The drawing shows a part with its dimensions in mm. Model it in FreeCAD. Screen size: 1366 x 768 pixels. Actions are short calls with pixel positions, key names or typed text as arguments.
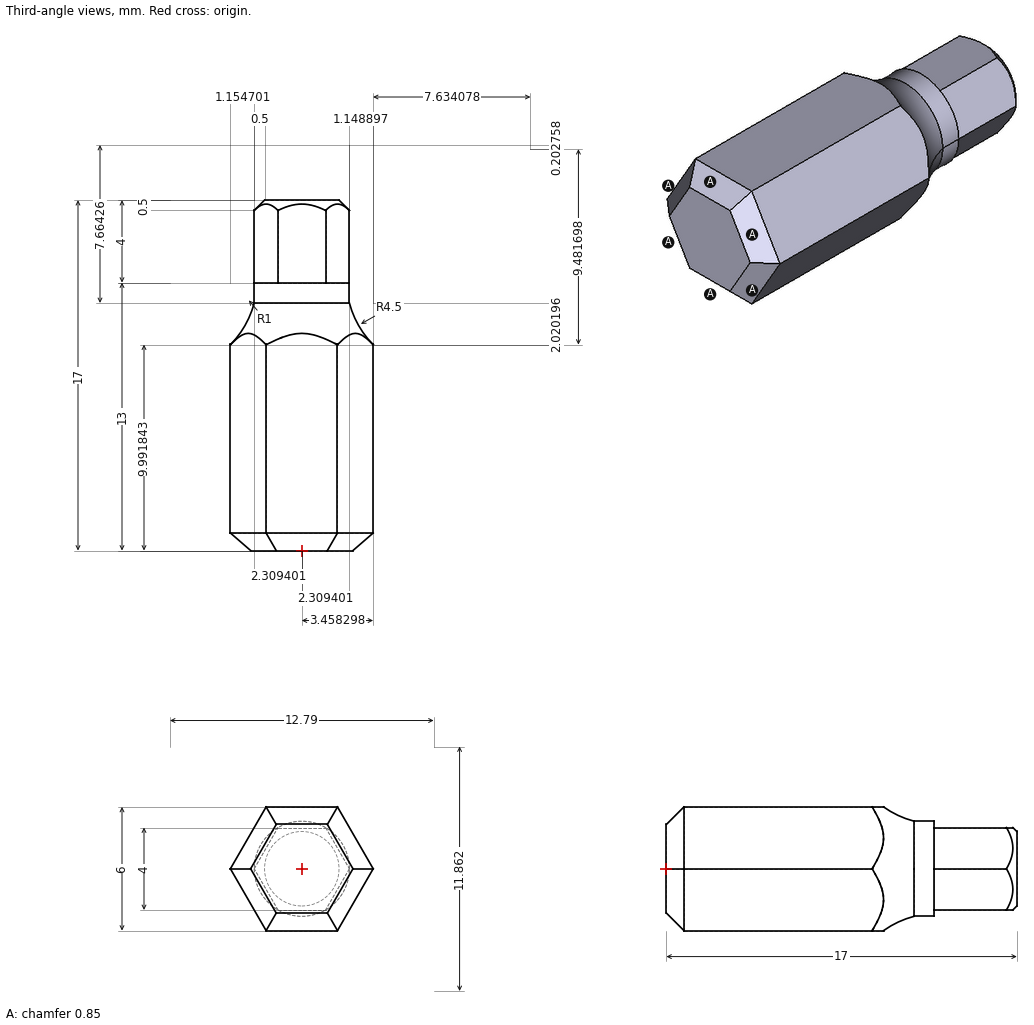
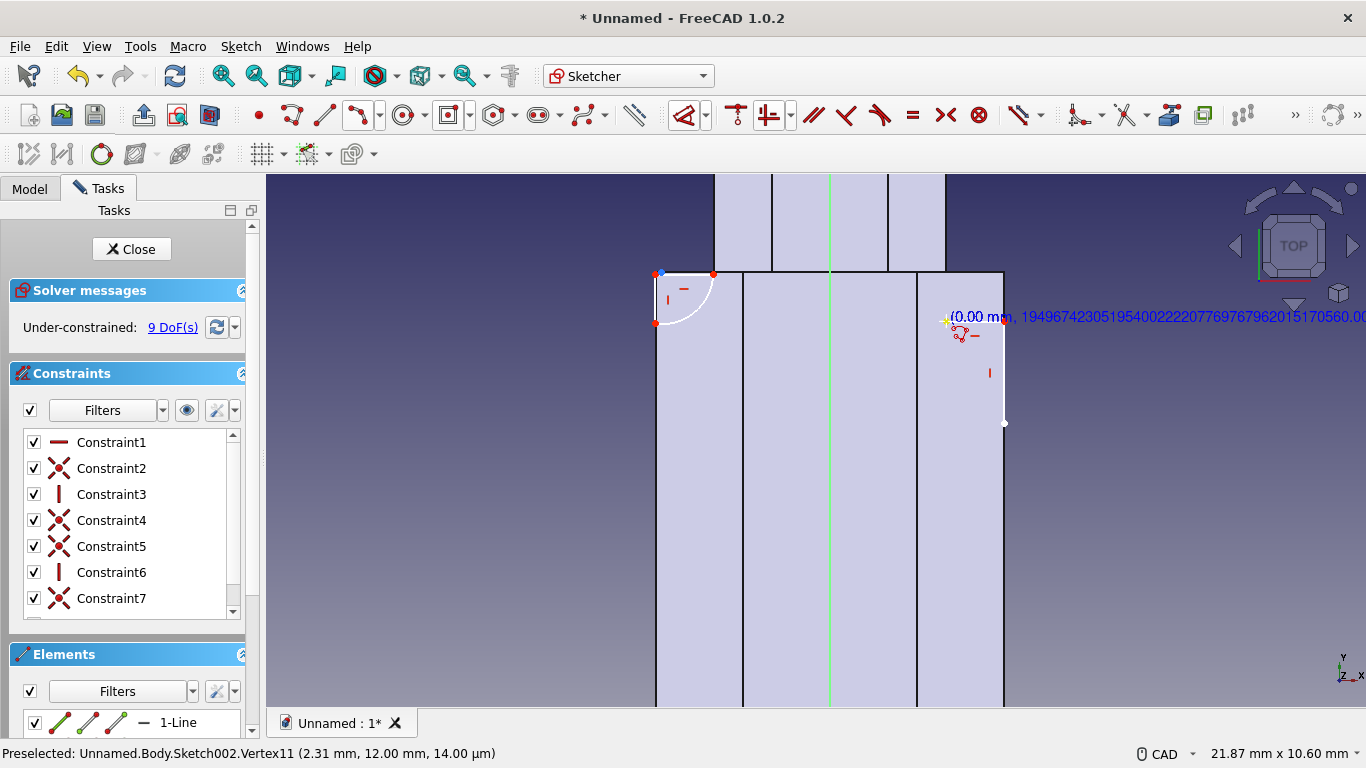
click(358, 116)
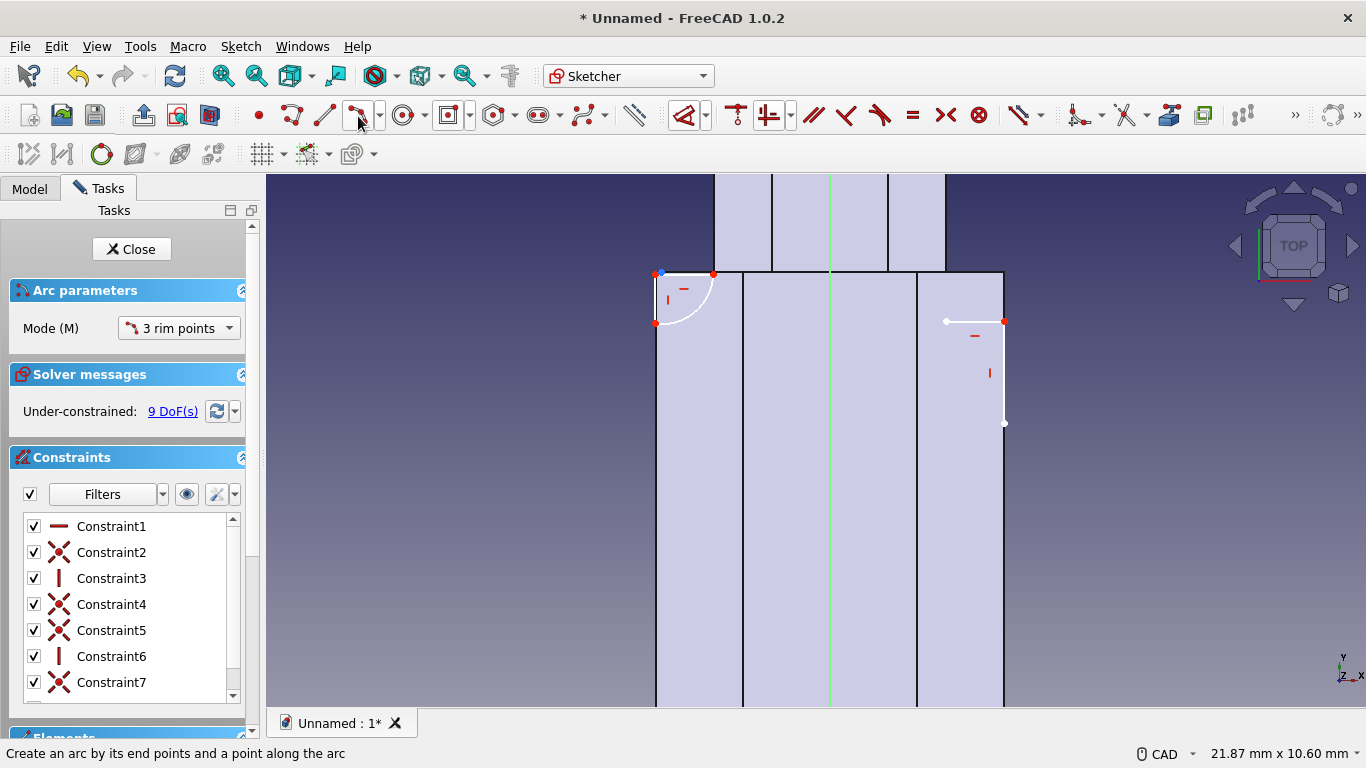
click(946, 322)
click(1004, 424)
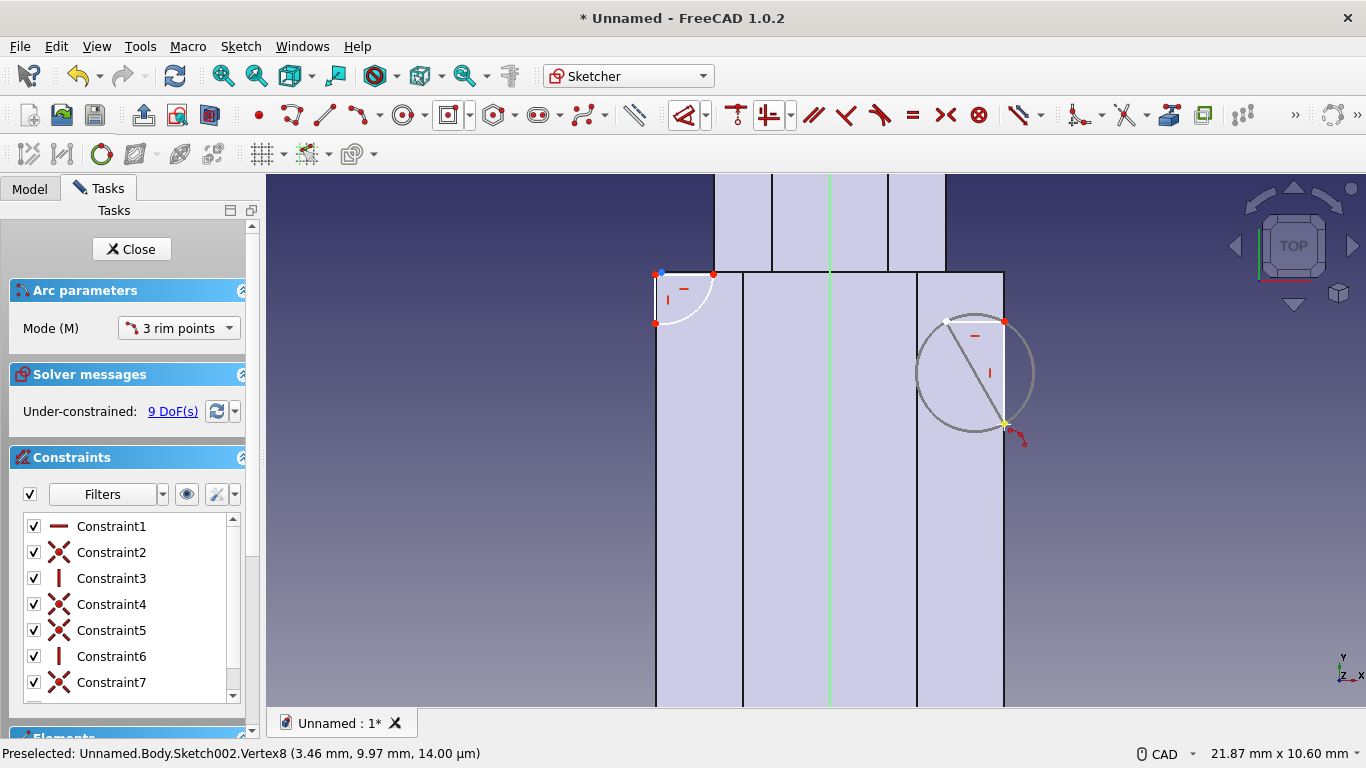
scroll(968, 376, up, 4)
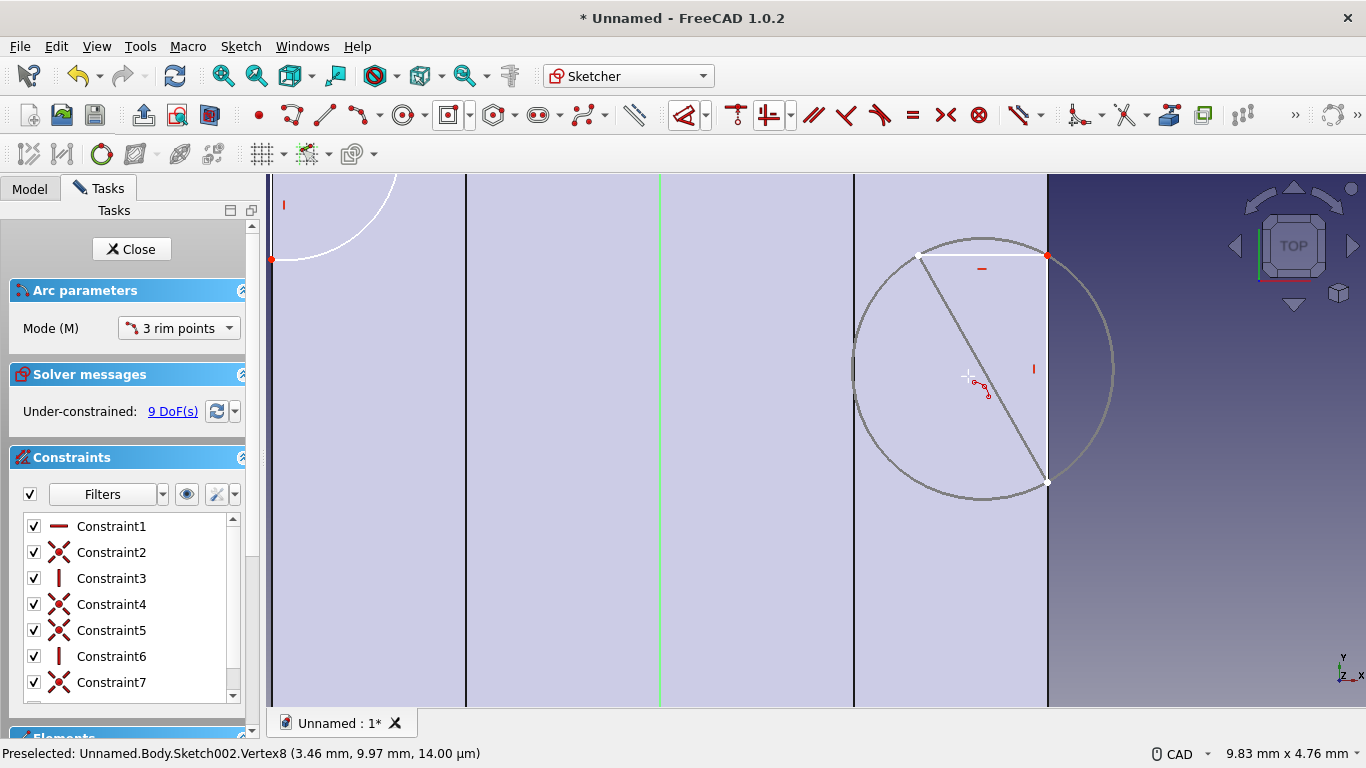
click(968, 376)
key(Escape)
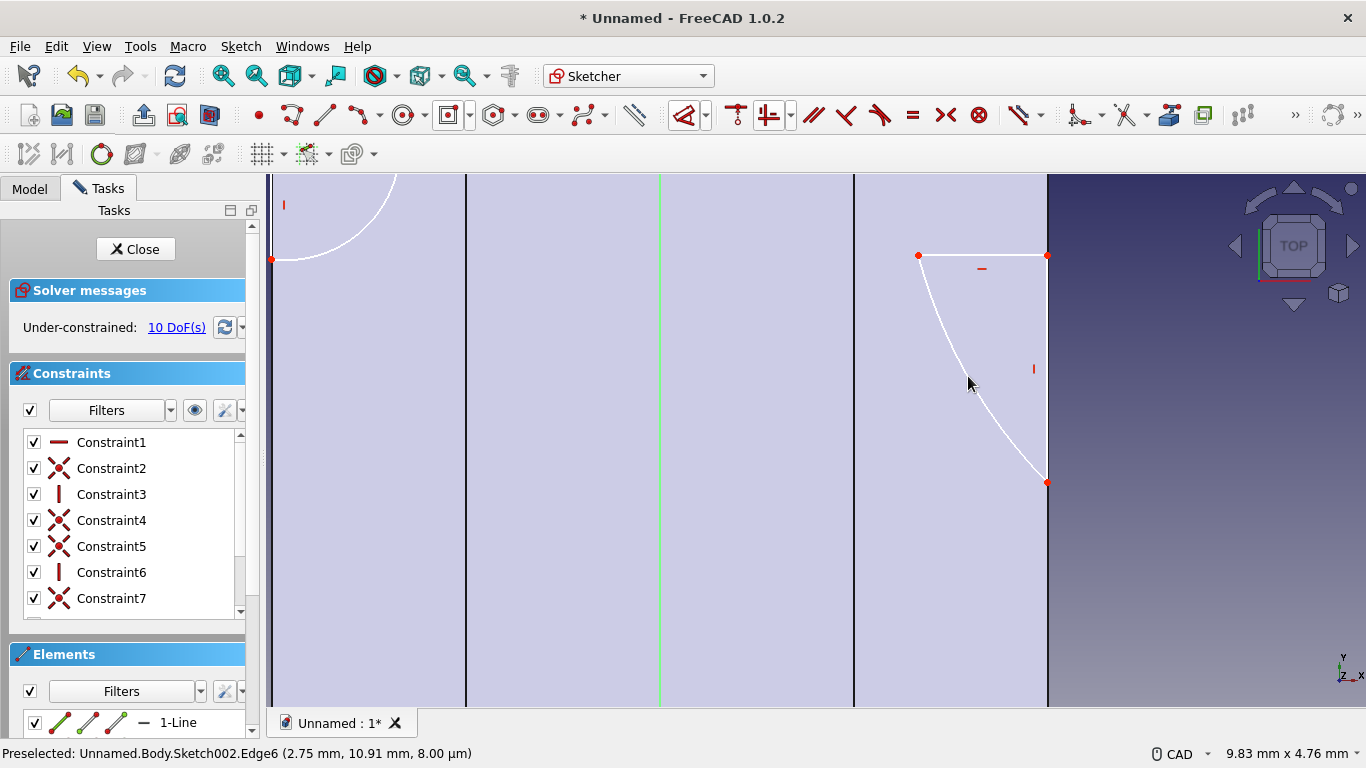
click(327, 252)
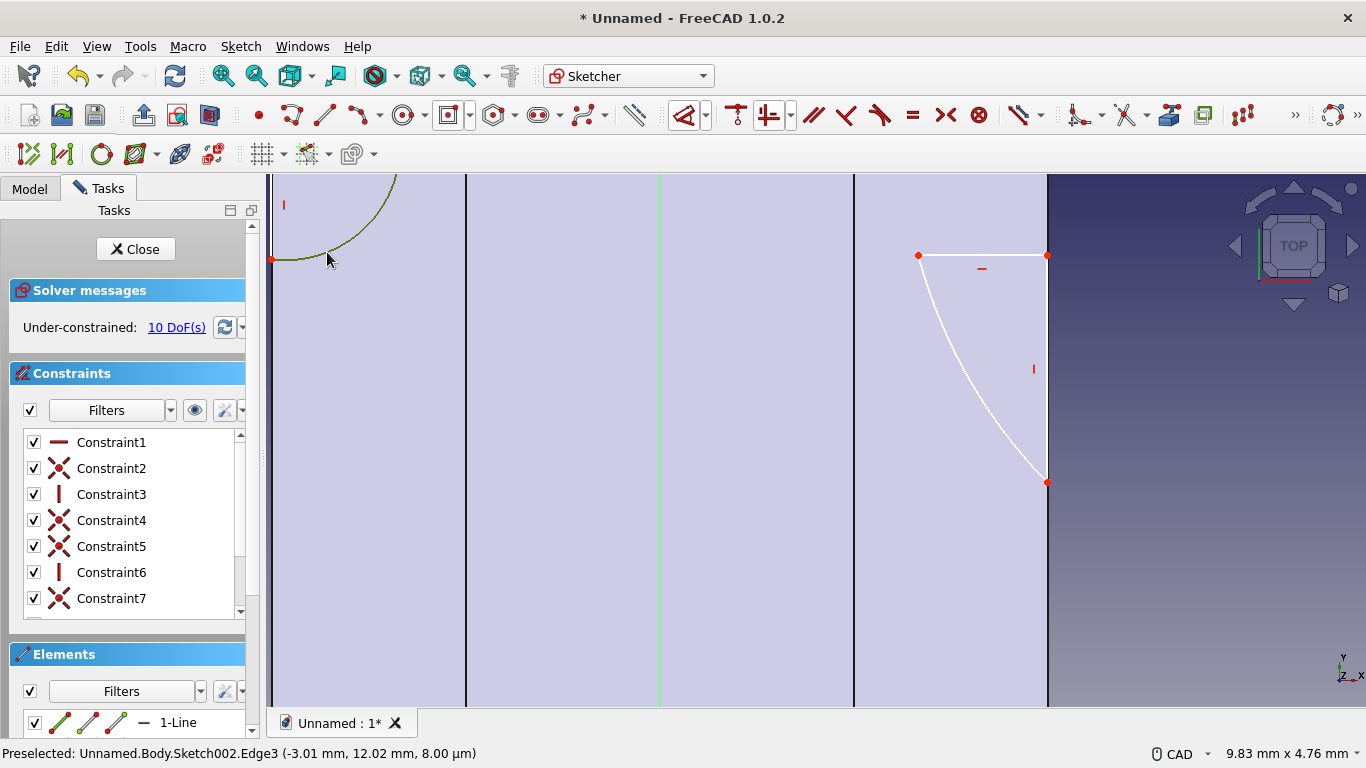
click(706, 116)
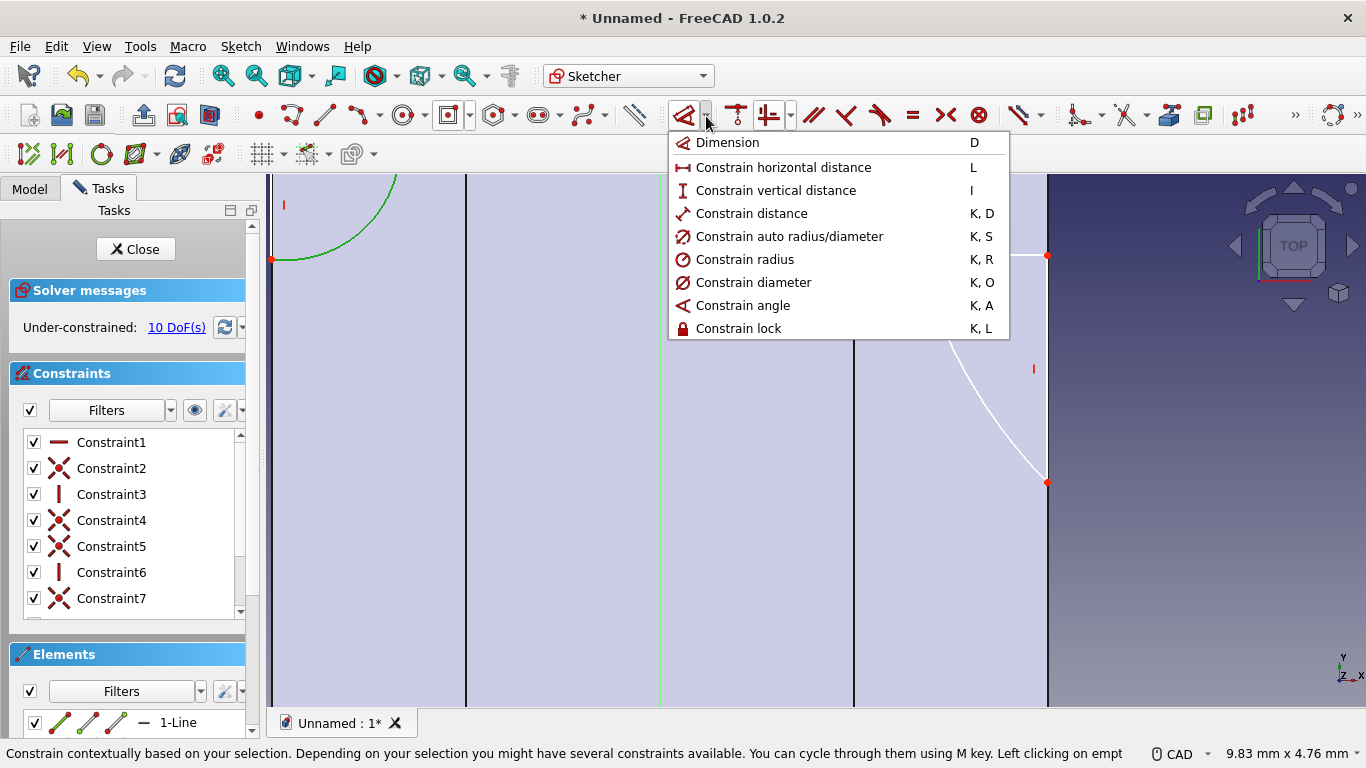
click(839, 260)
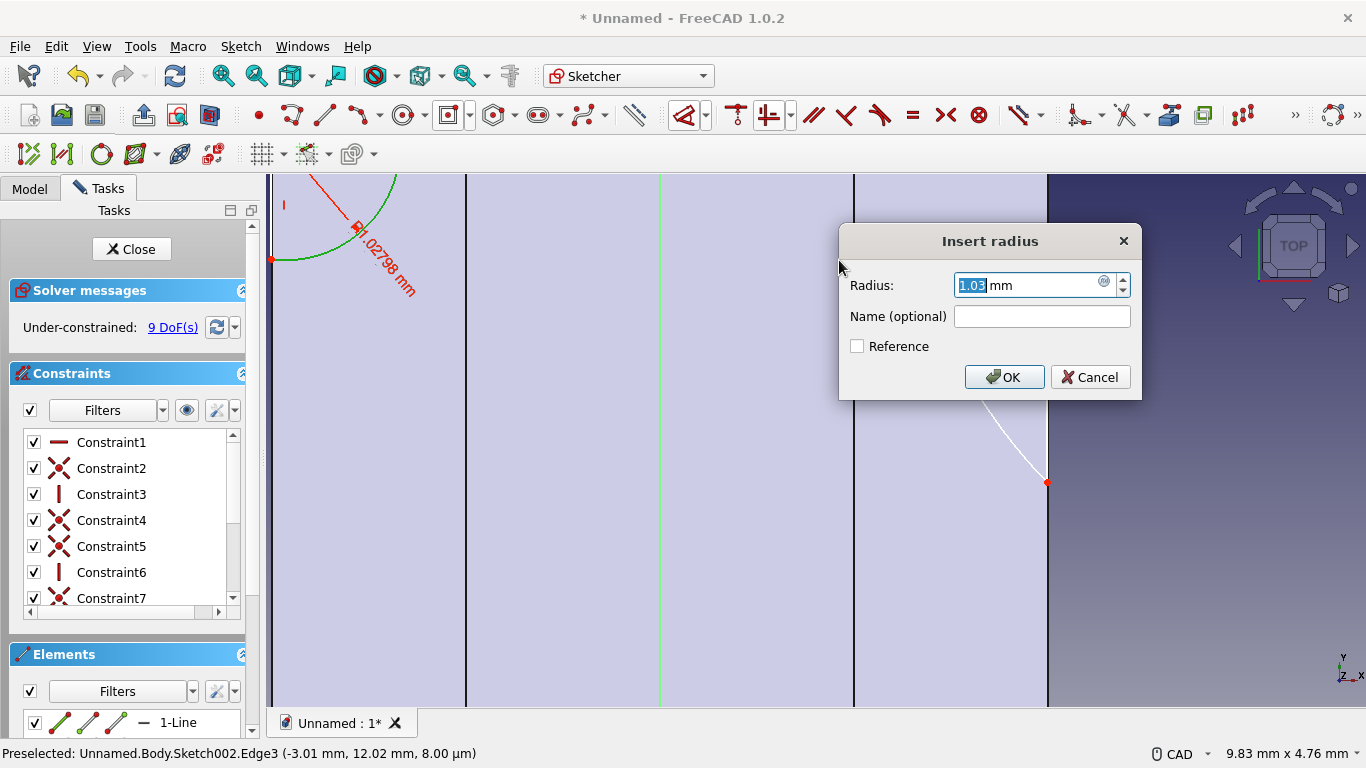
text(1)
key(Return)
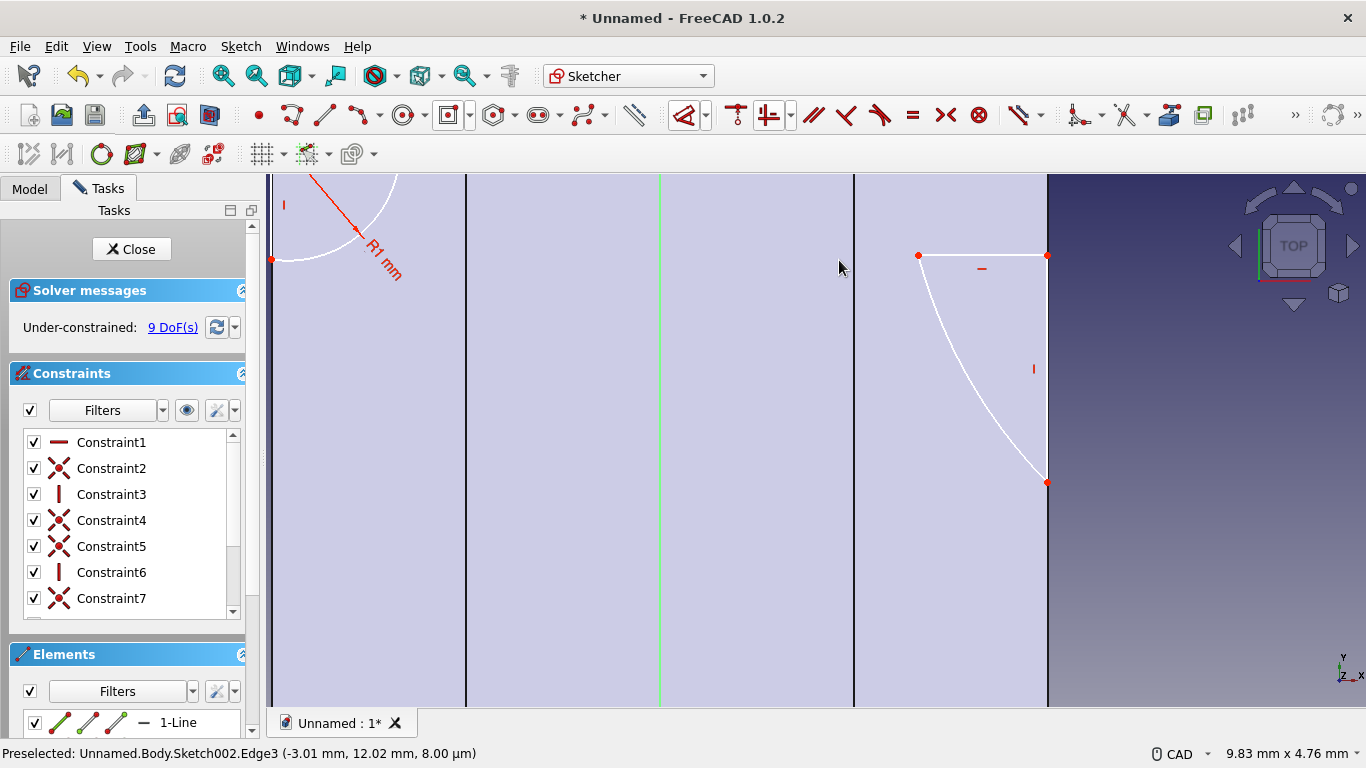
scroll(776, 300, down, 7)